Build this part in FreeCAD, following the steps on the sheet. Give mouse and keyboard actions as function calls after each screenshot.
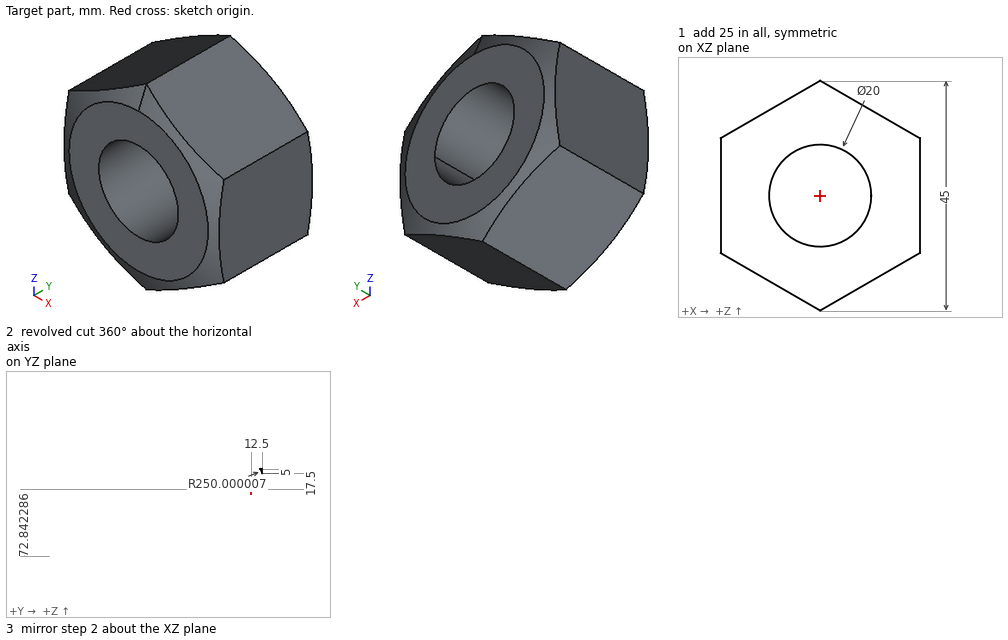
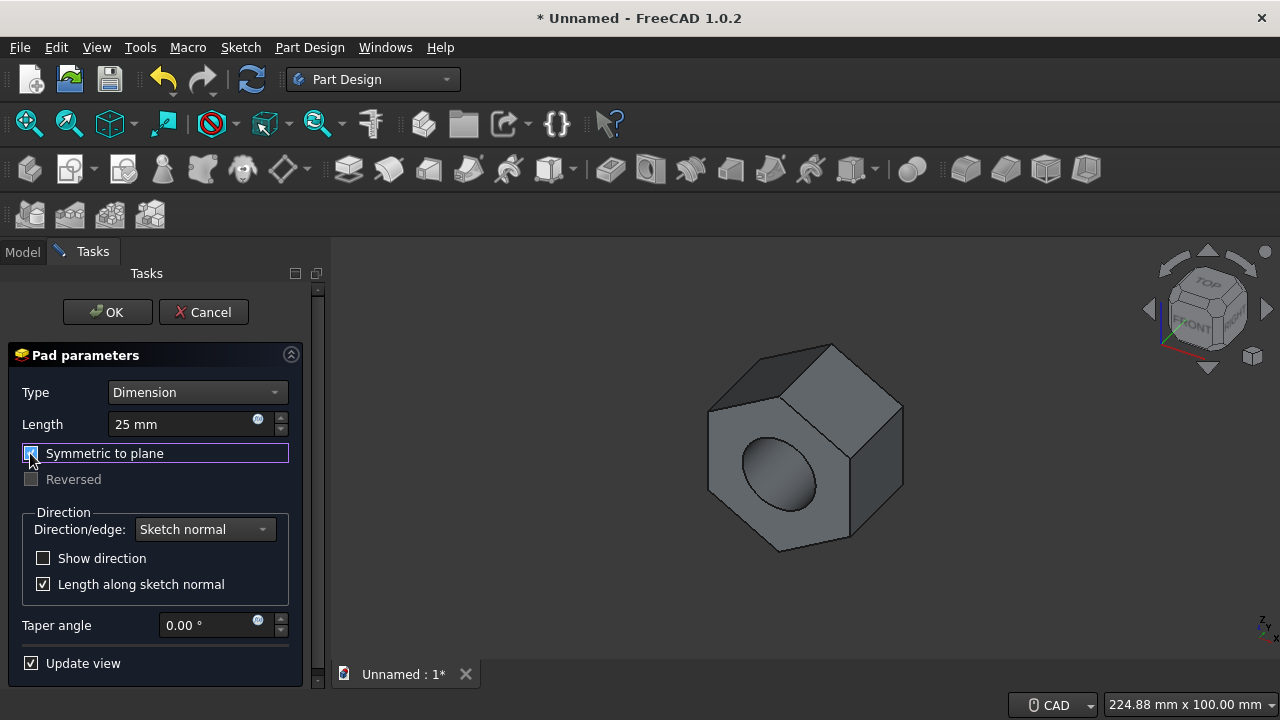
click(108, 312)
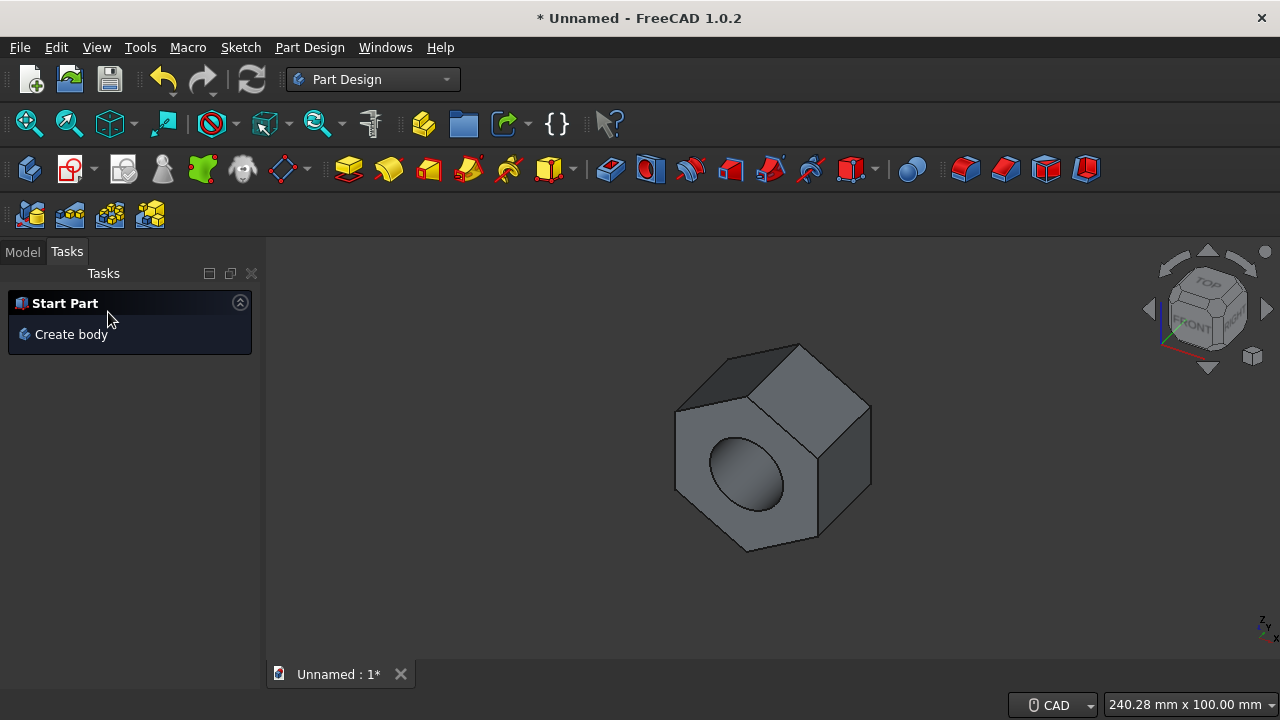
click(70, 170)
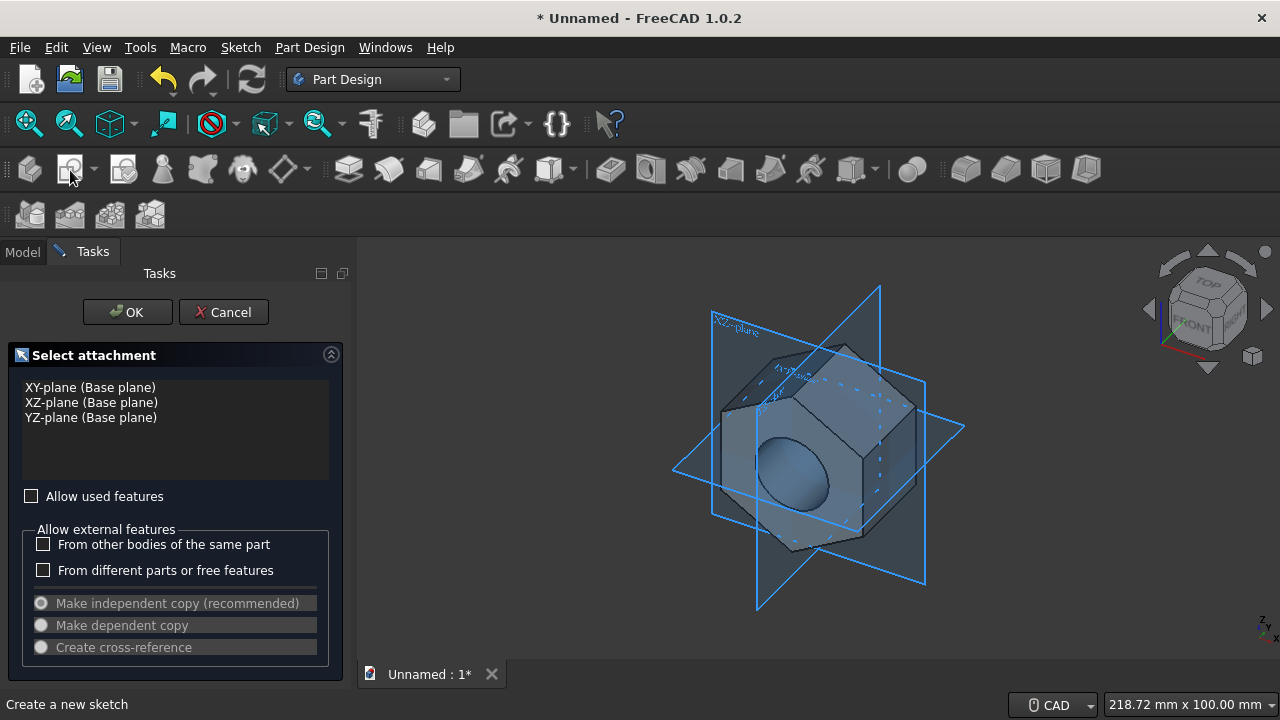
click(82, 418)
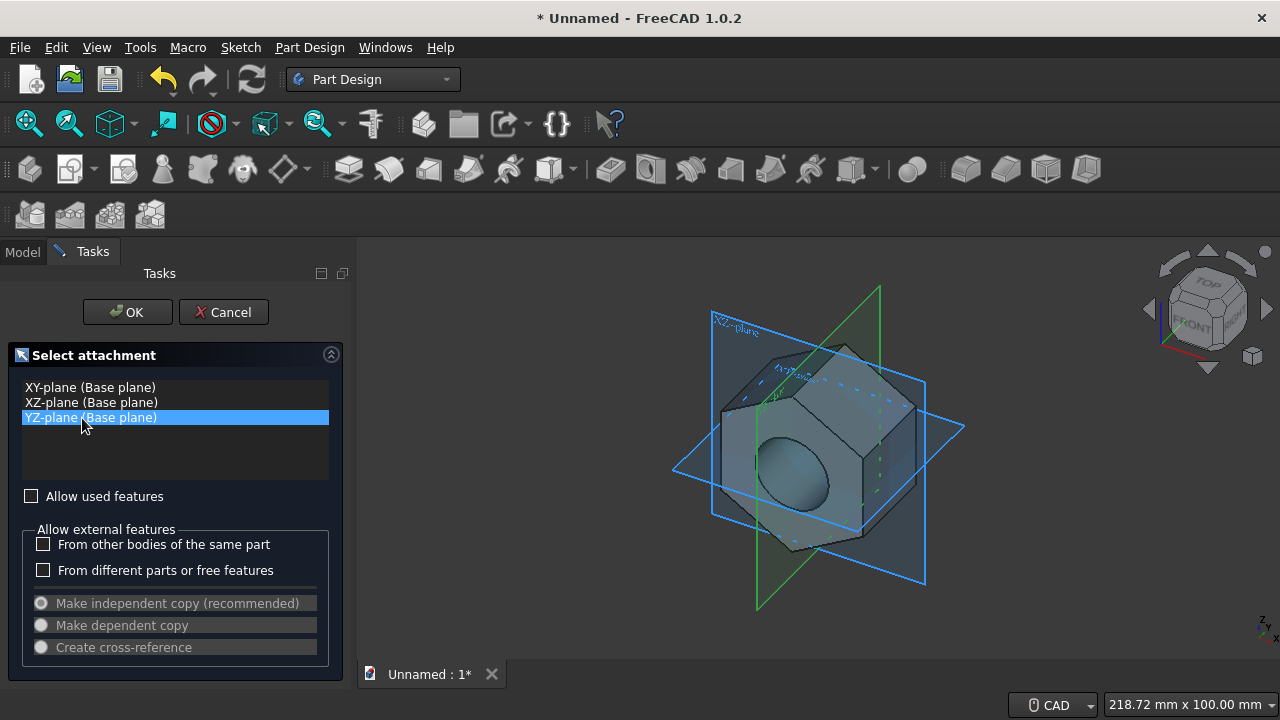
click(128, 312)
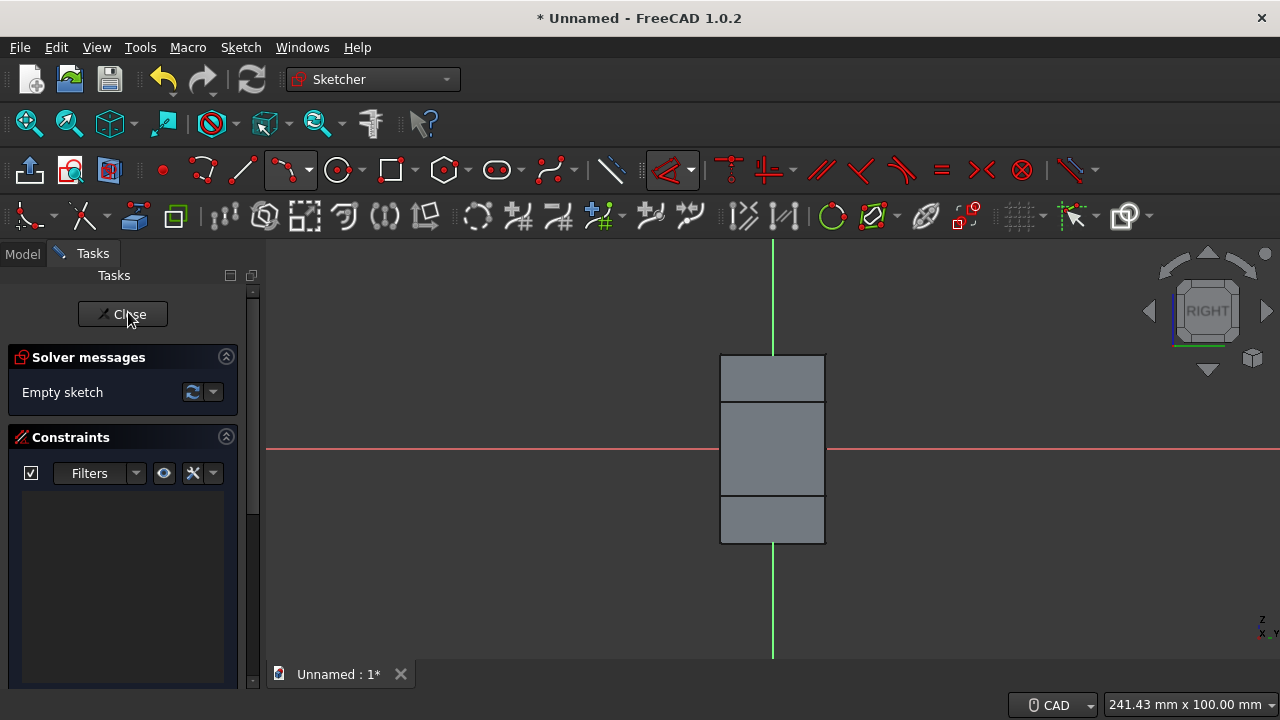
key(q)
key(s)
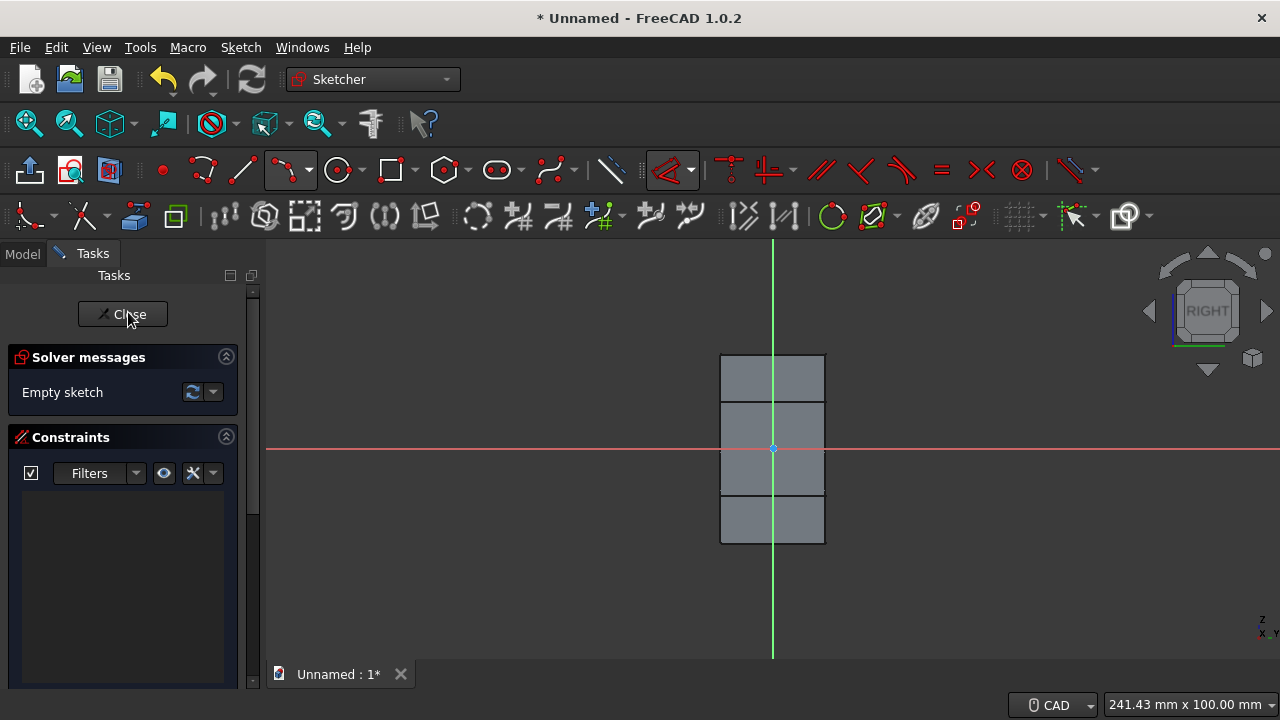
scroll(831, 358, up, 13)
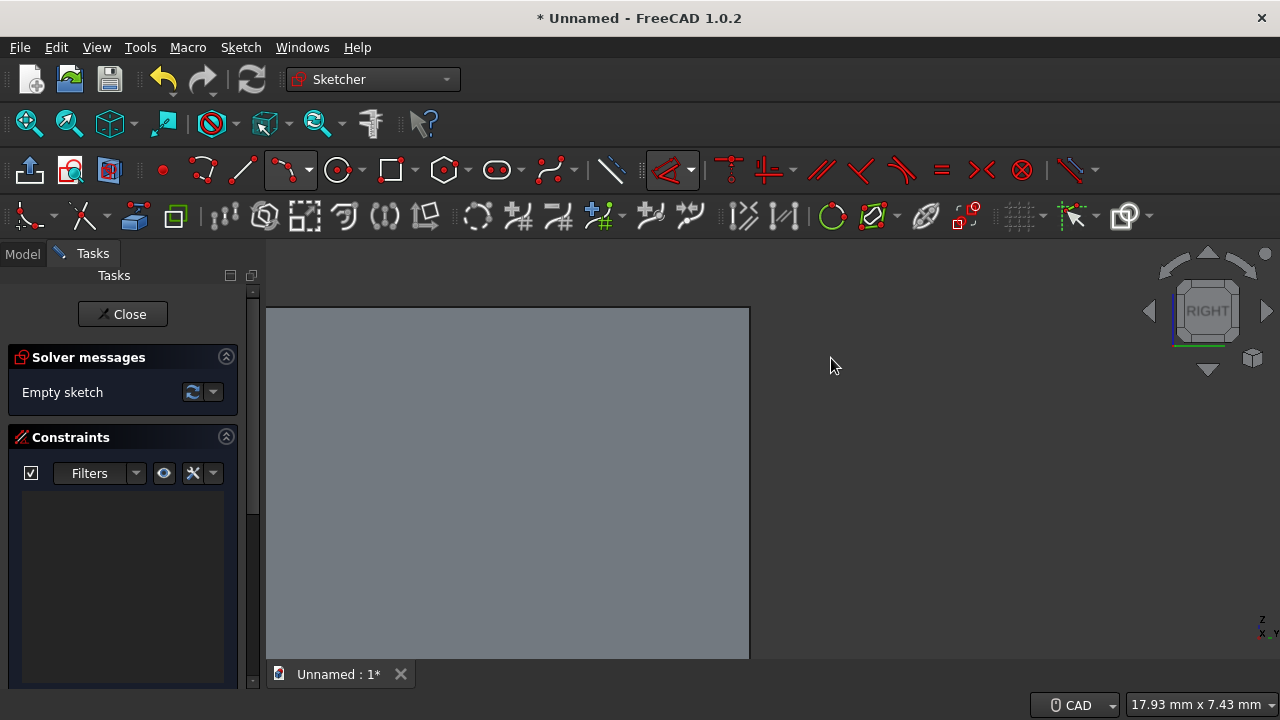
click(204, 170)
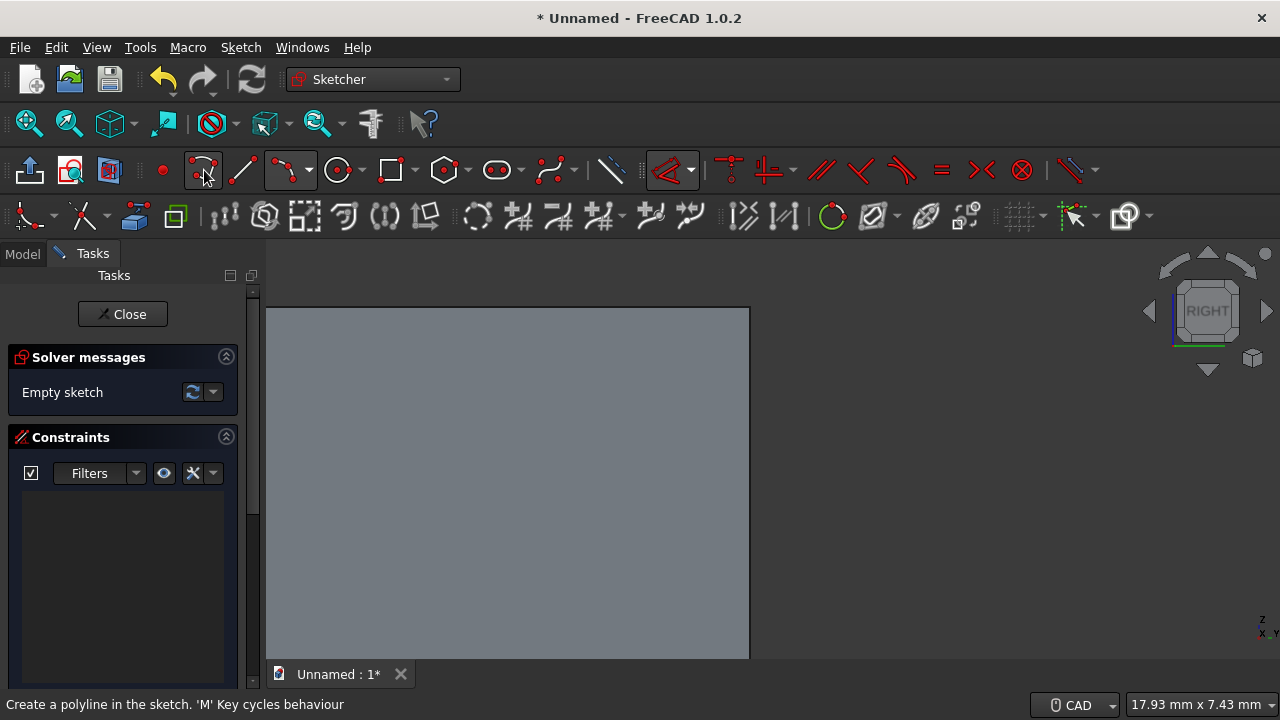
click(750, 590)
click(750, 307)
click(637, 307)
right_click(637, 307)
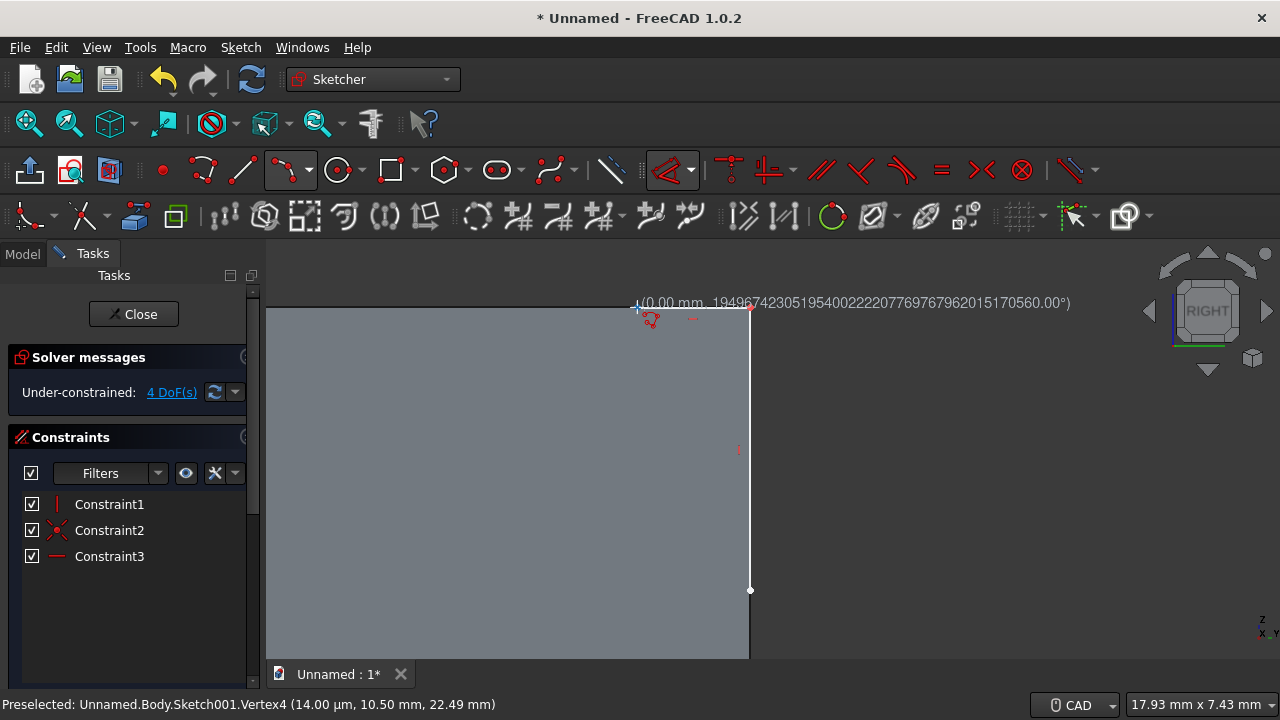
click(284, 170)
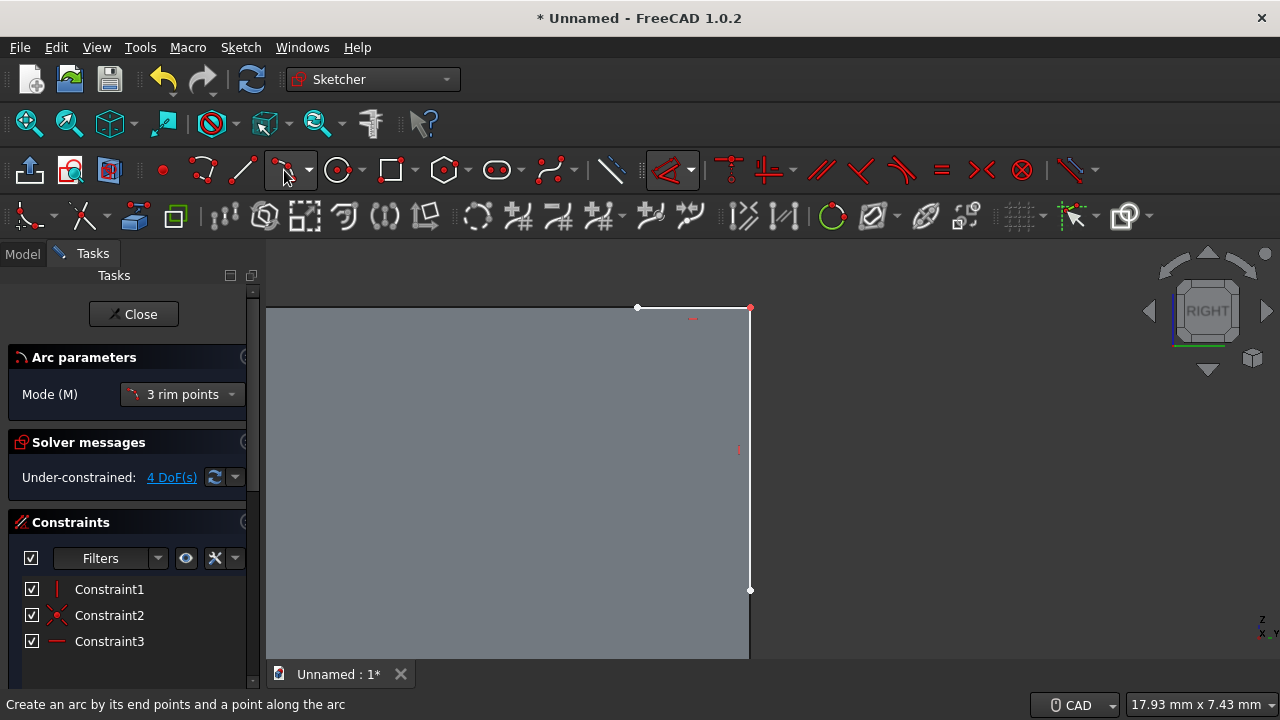
click(637, 308)
click(750, 591)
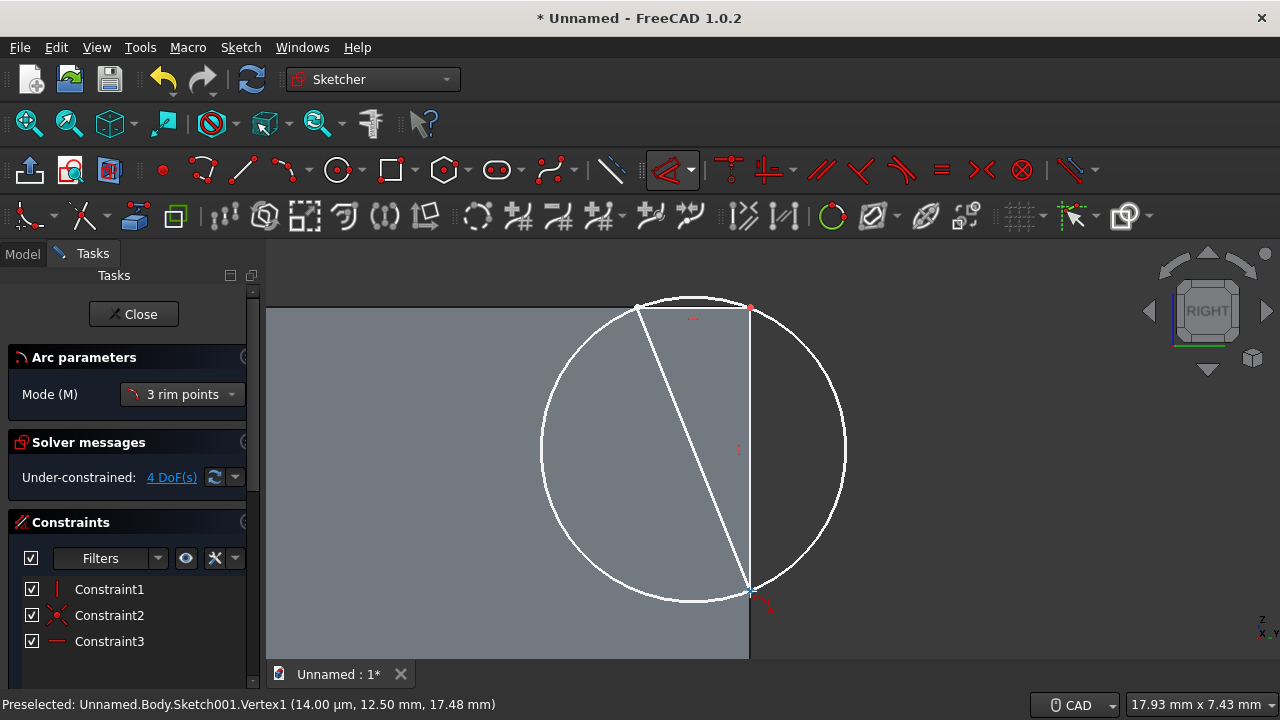
scroll(694, 448, up, 15)